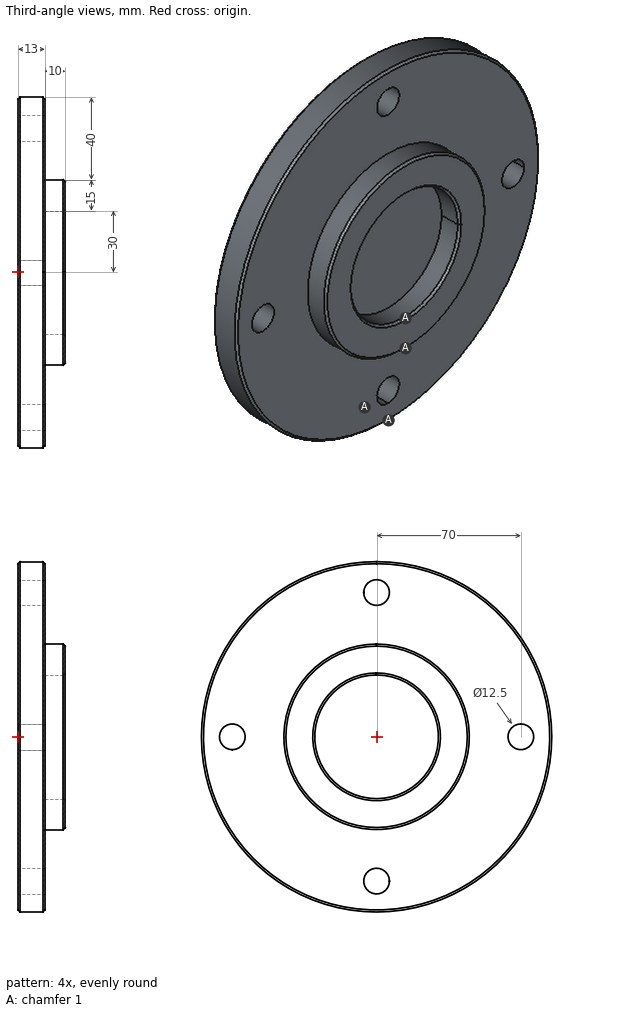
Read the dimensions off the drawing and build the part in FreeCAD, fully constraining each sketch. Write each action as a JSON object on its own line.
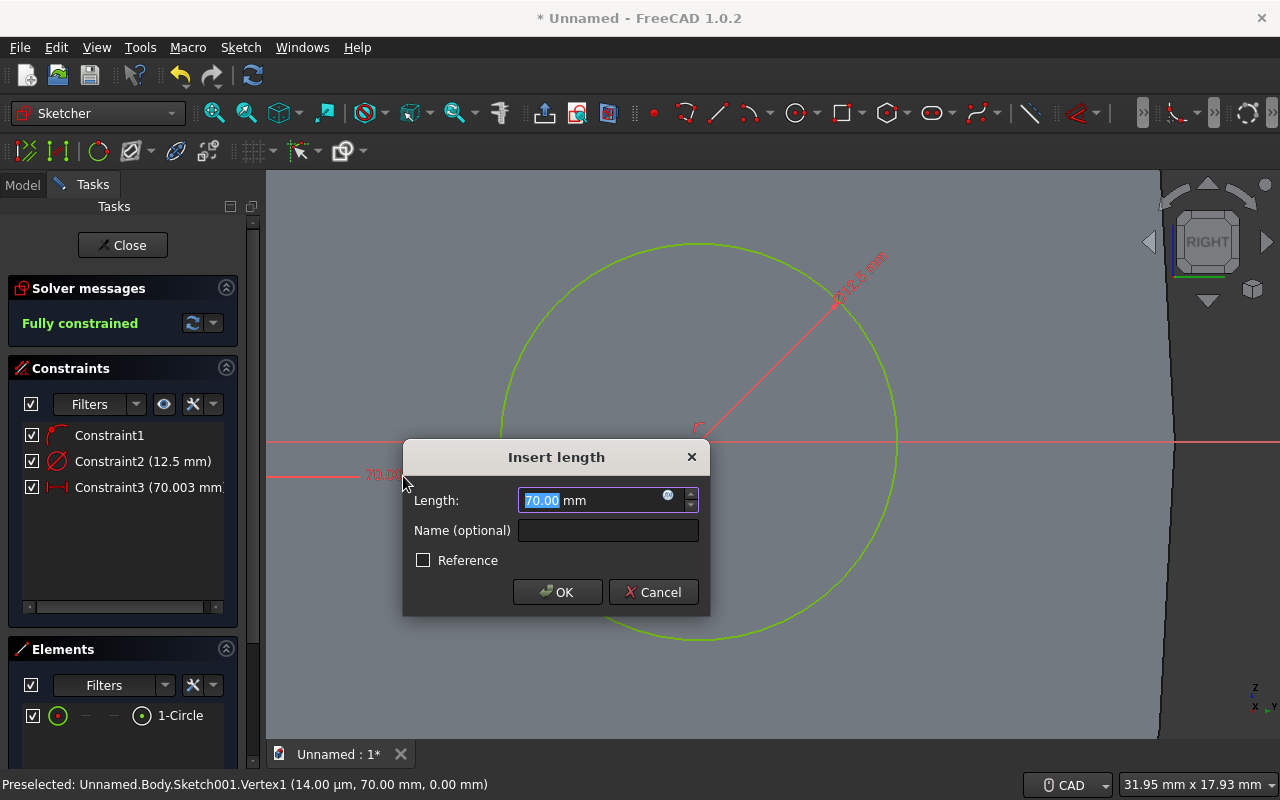
{"action": "type", "text": "70"}
{"action": "key", "text": "Return"}
{"action": "key", "text": "Escape"}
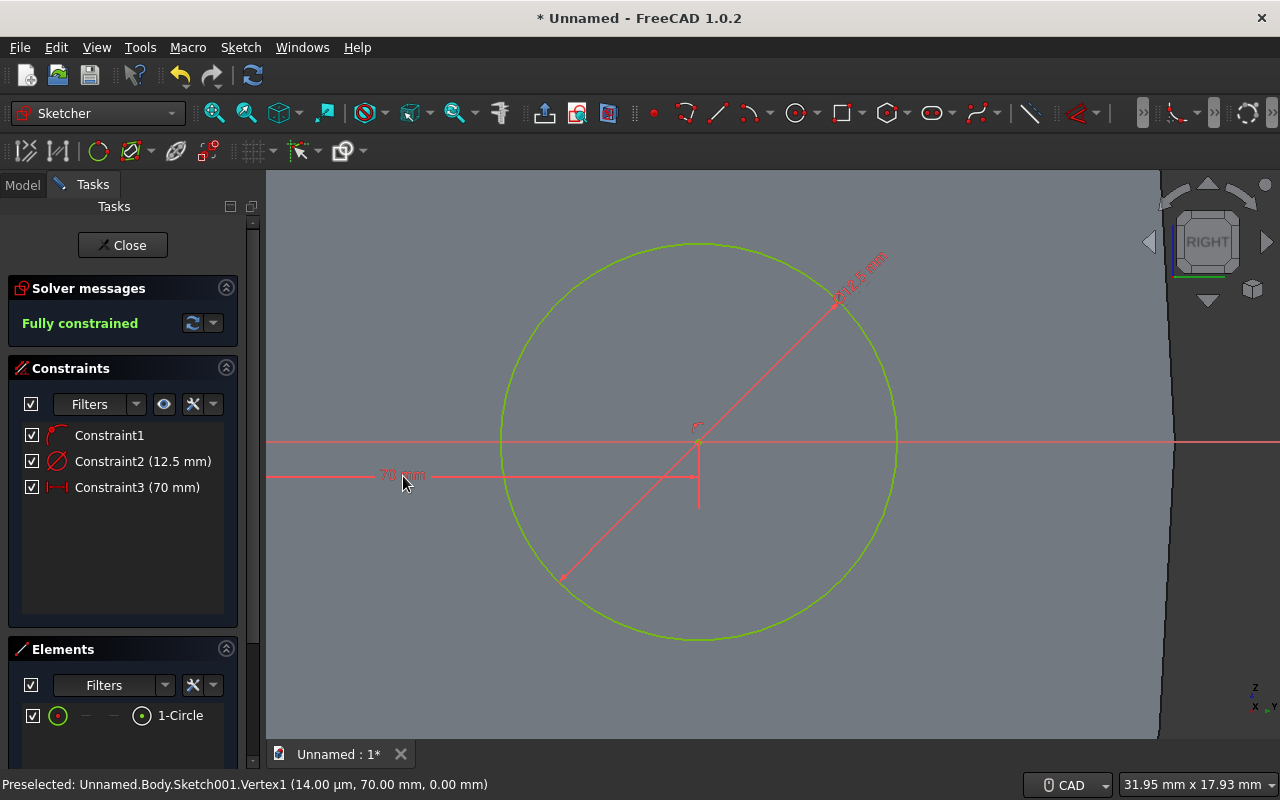
{"action": "left_click", "coordinate": [123, 245]}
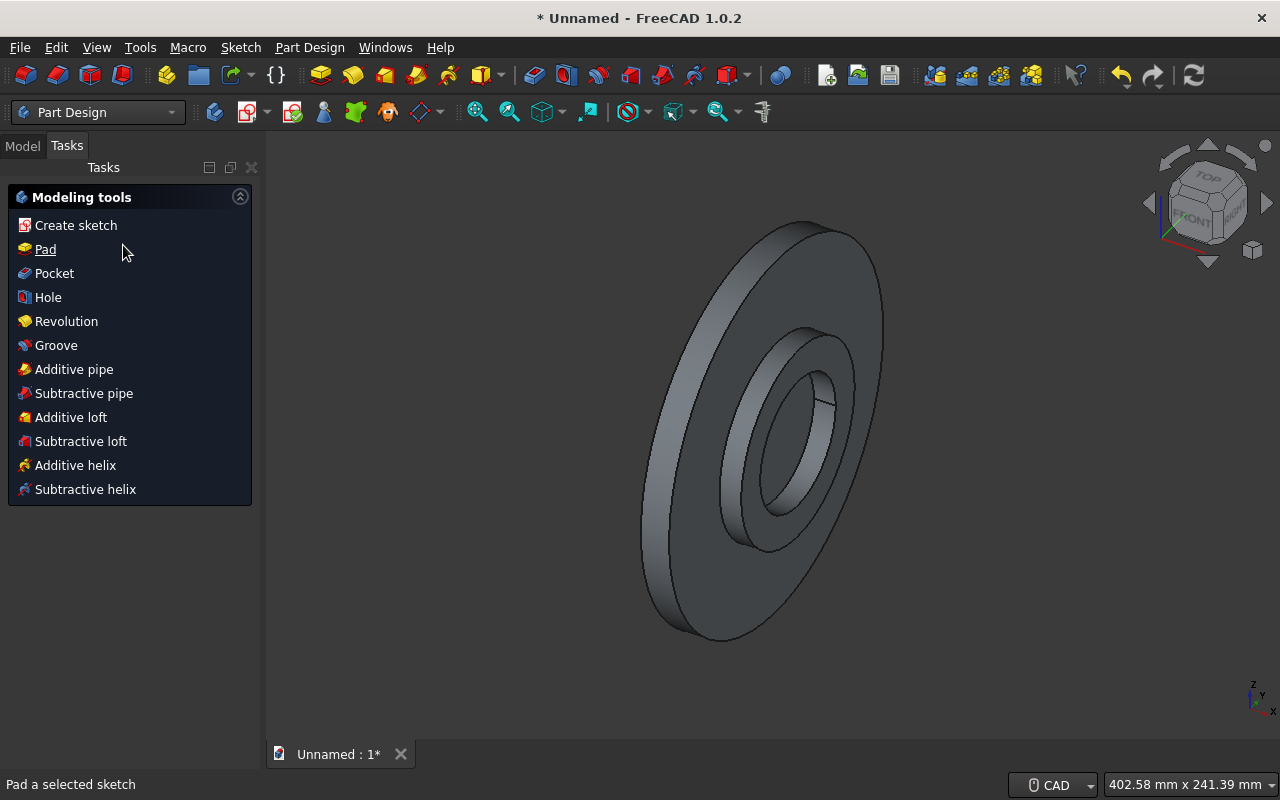
{"action": "left_click", "coordinate": [536, 76]}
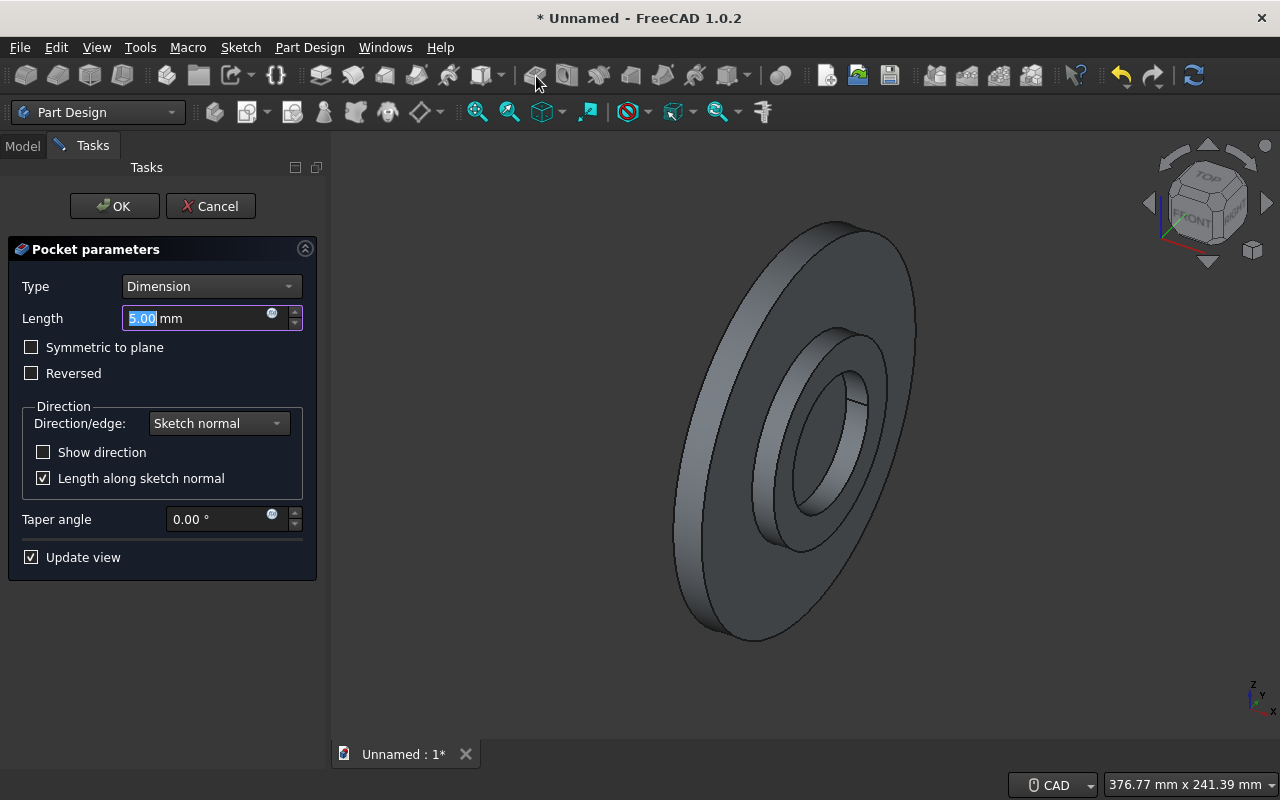
{"action": "left_click", "coordinate": [212, 286]}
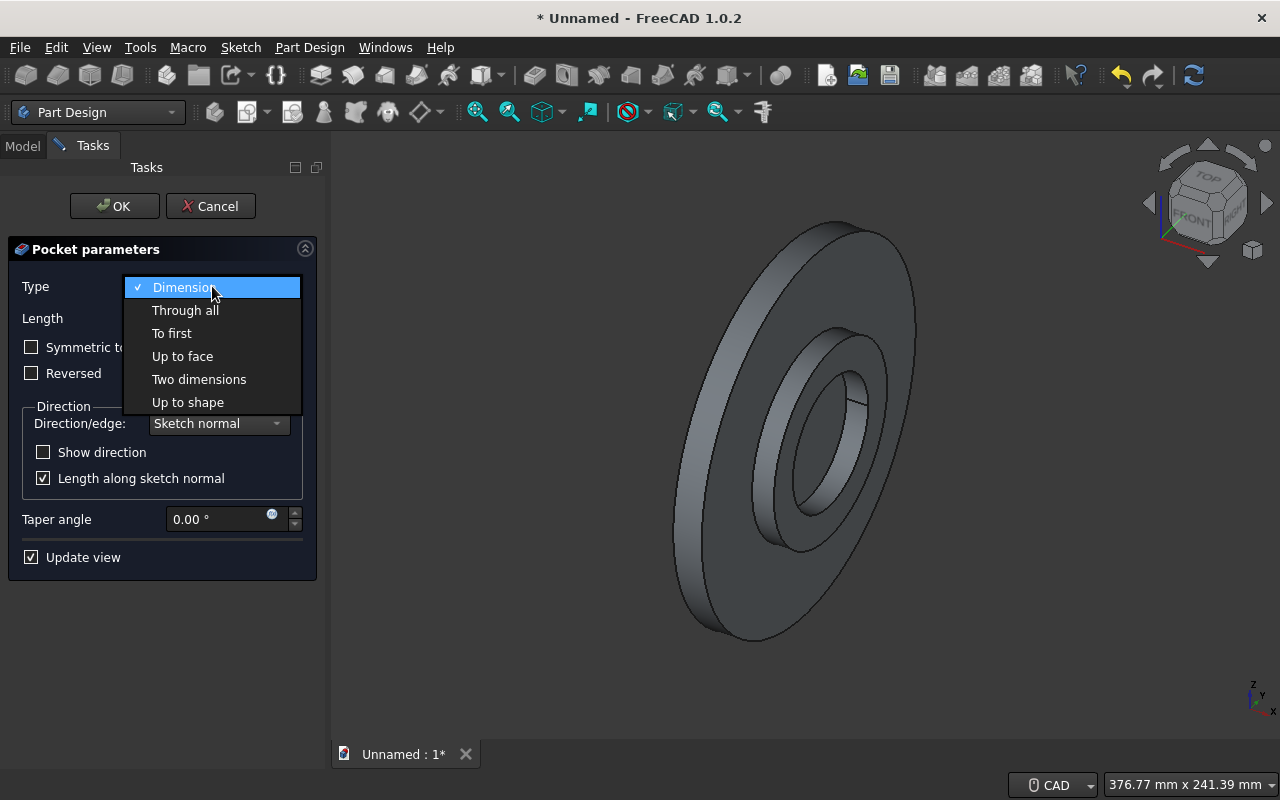
{"action": "left_click", "coordinate": [212, 310]}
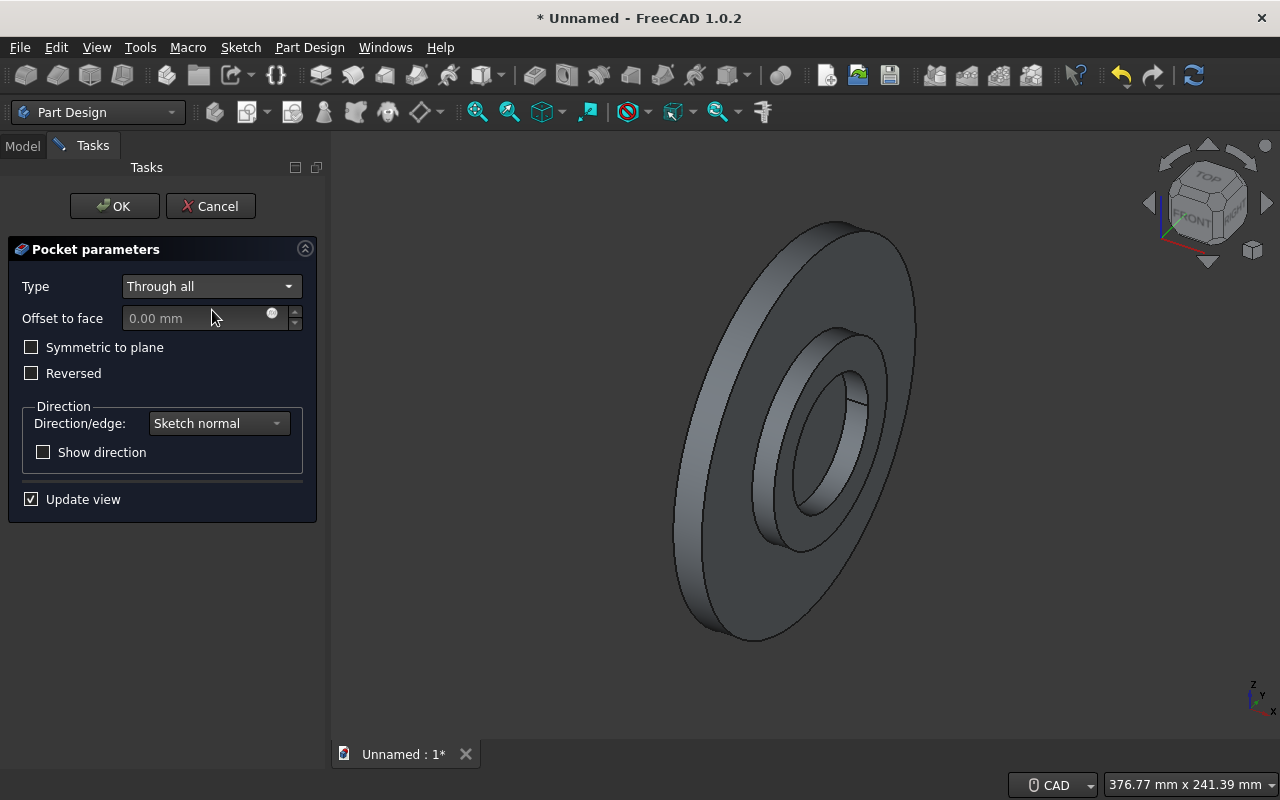
{"action": "left_click", "coordinate": [30, 373]}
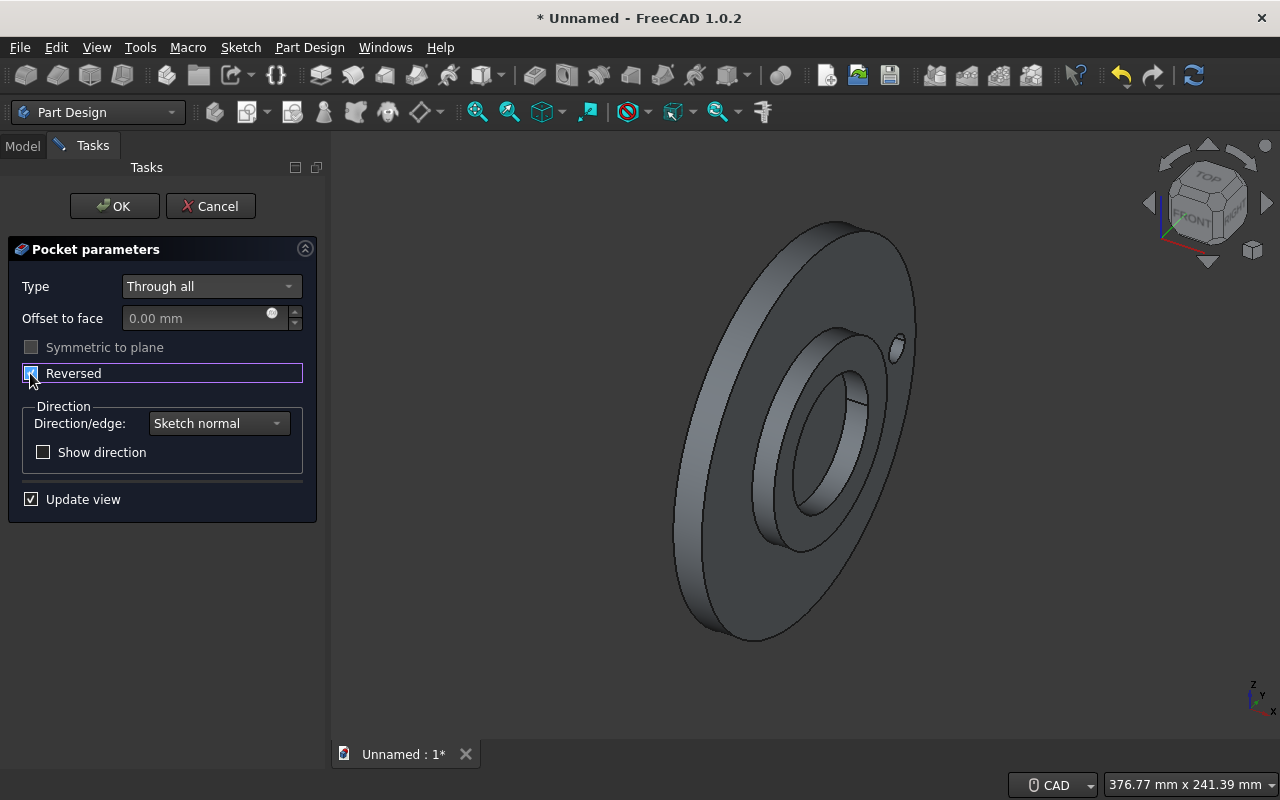
{"action": "left_click", "coordinate": [115, 206]}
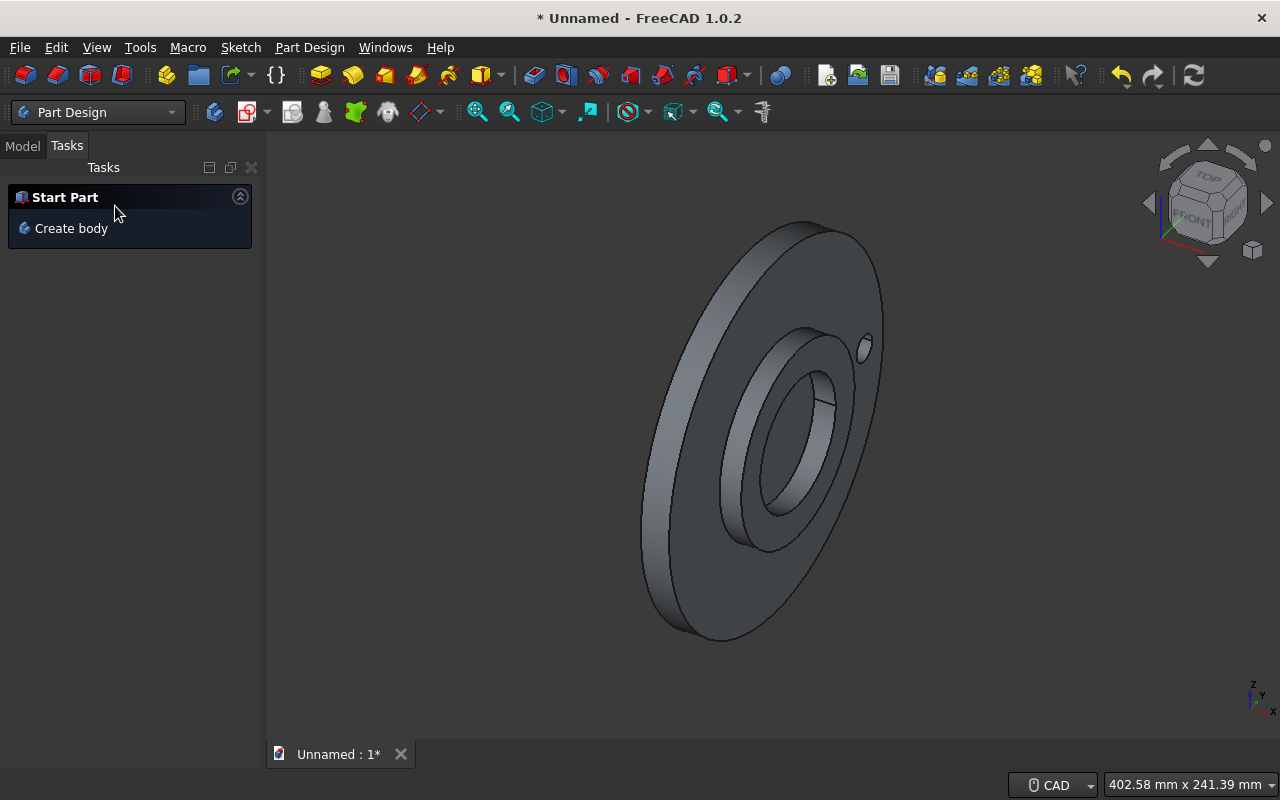
{"action": "left_click", "coordinate": [23, 145]}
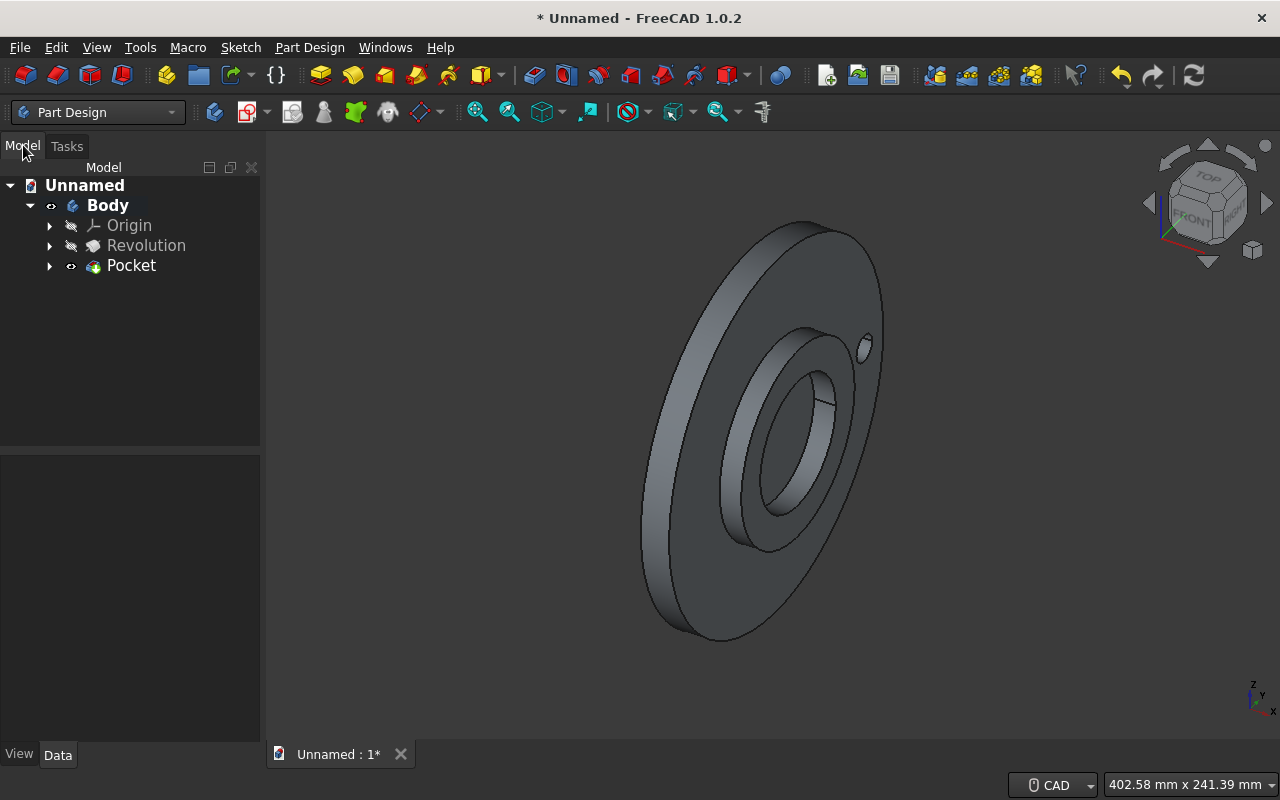
{"action": "left_click", "coordinate": [116, 266]}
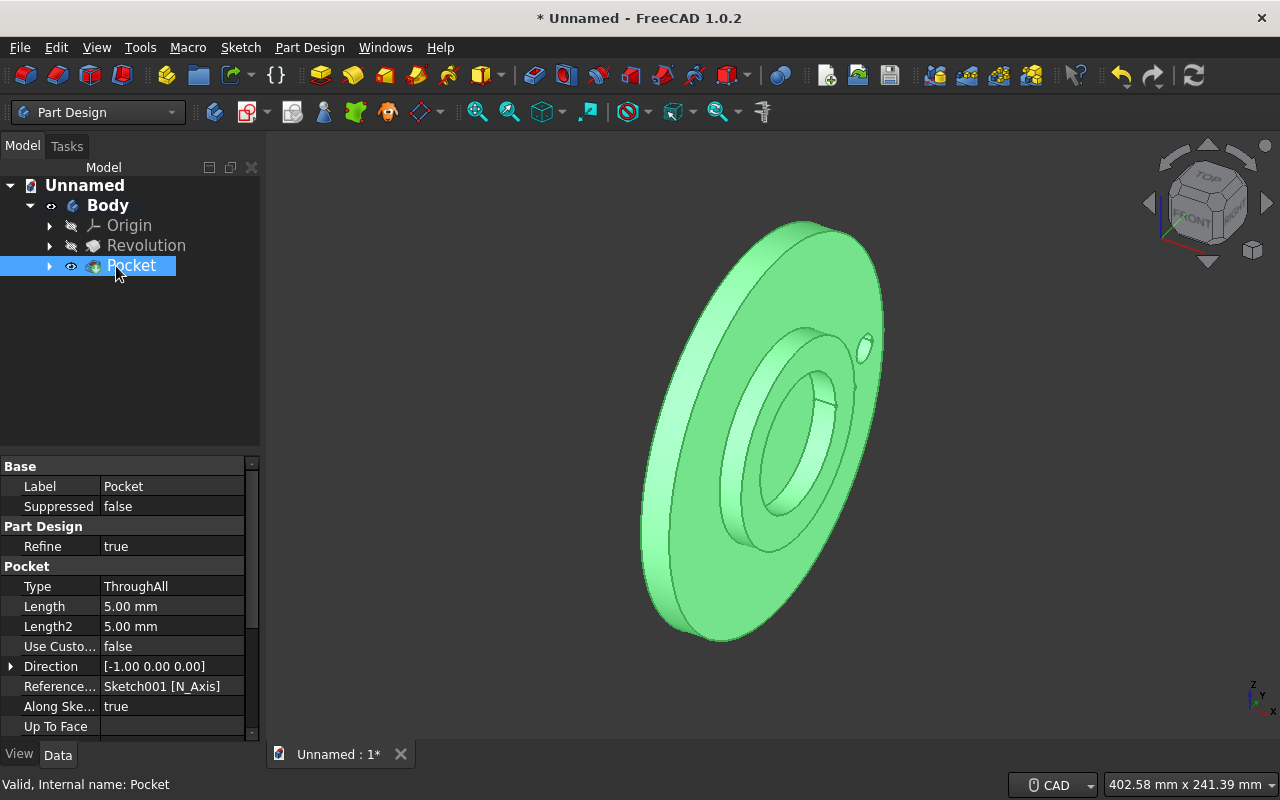
{"action": "left_click", "coordinate": [1000, 76]}